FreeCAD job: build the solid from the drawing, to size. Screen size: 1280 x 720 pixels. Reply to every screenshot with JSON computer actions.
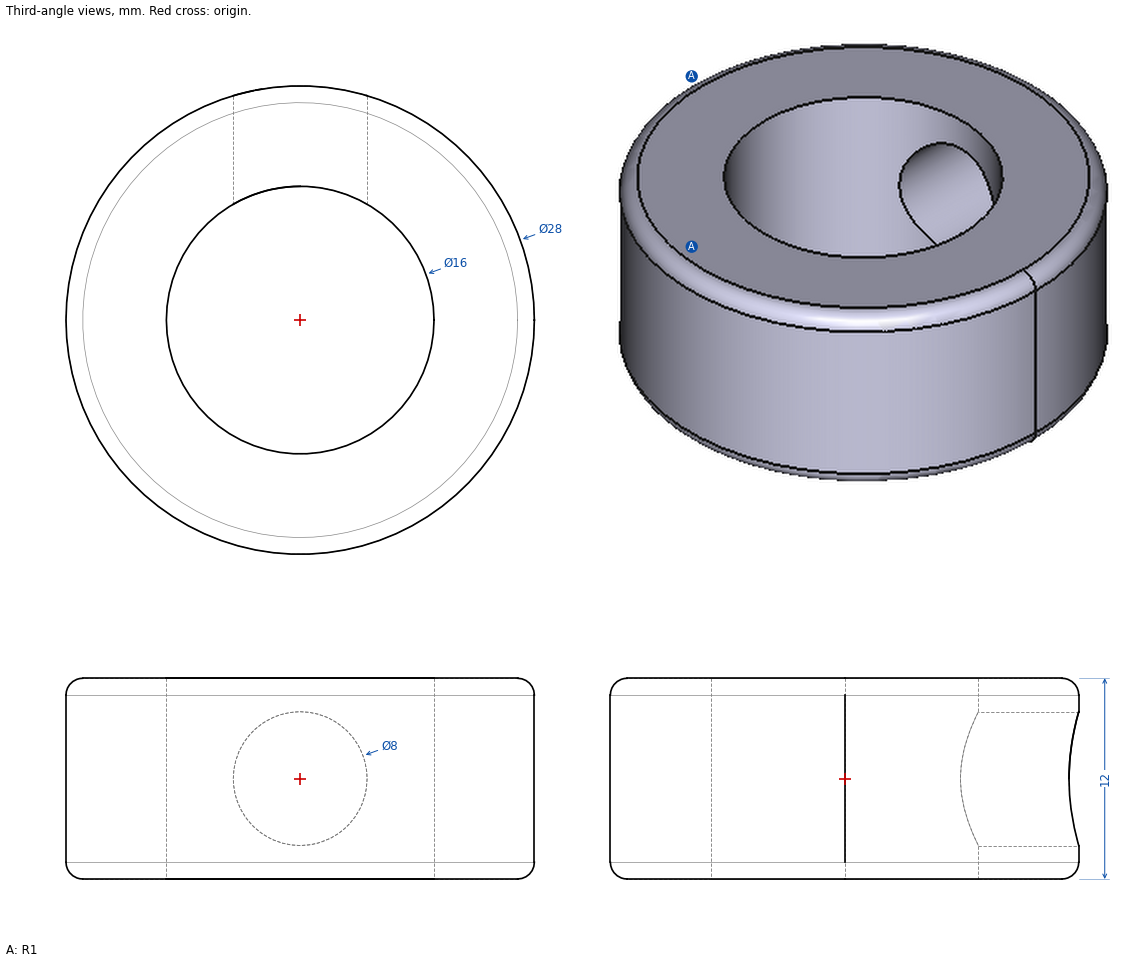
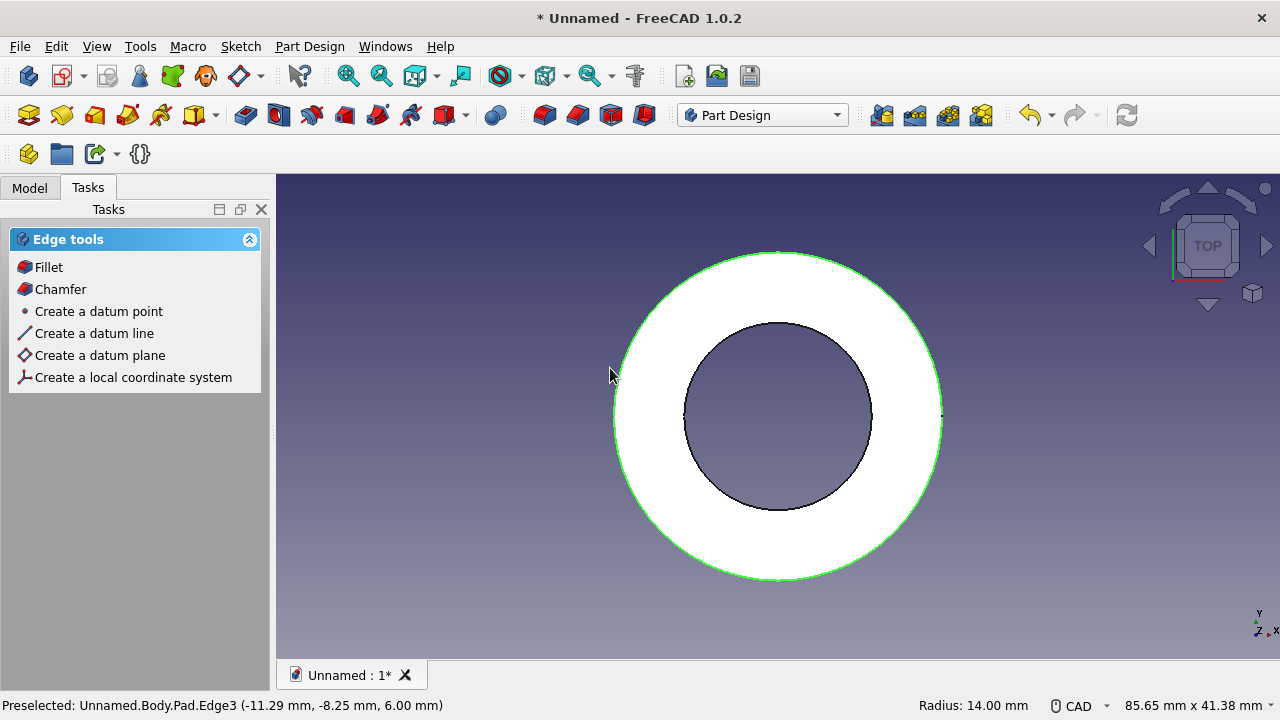
{"action": "key", "text": "1"}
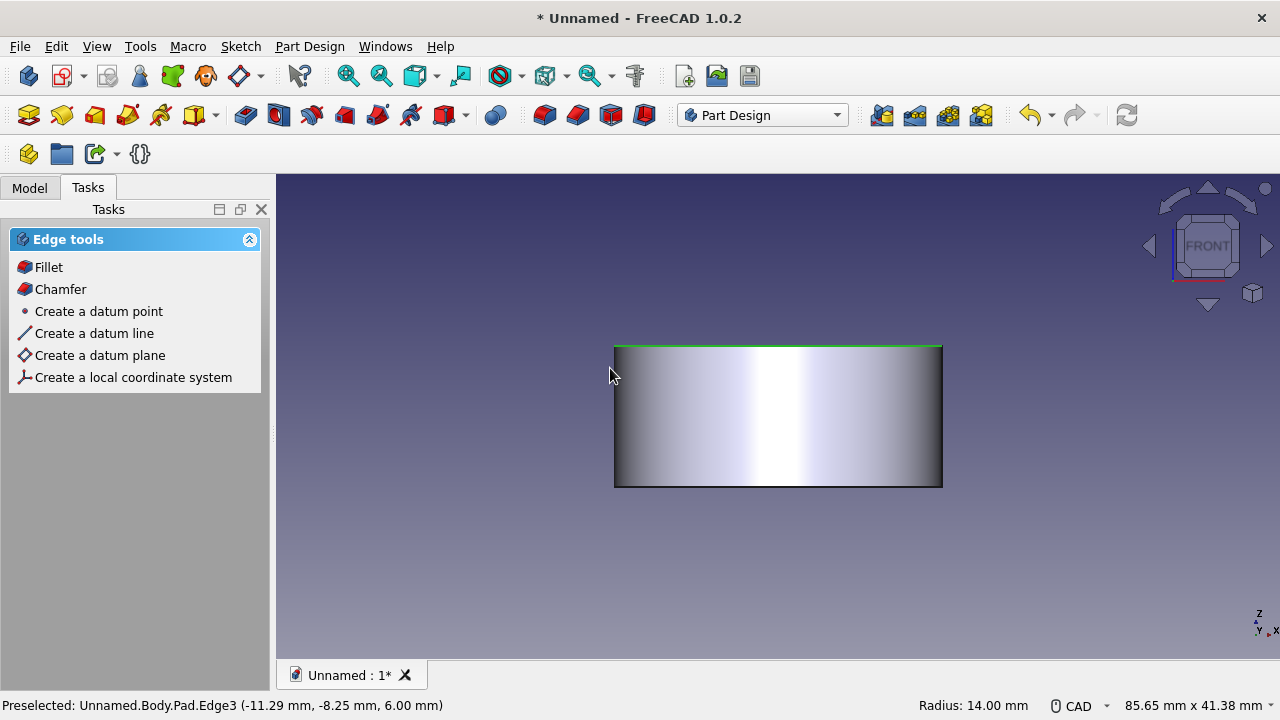
{"action": "key", "text": "v f"}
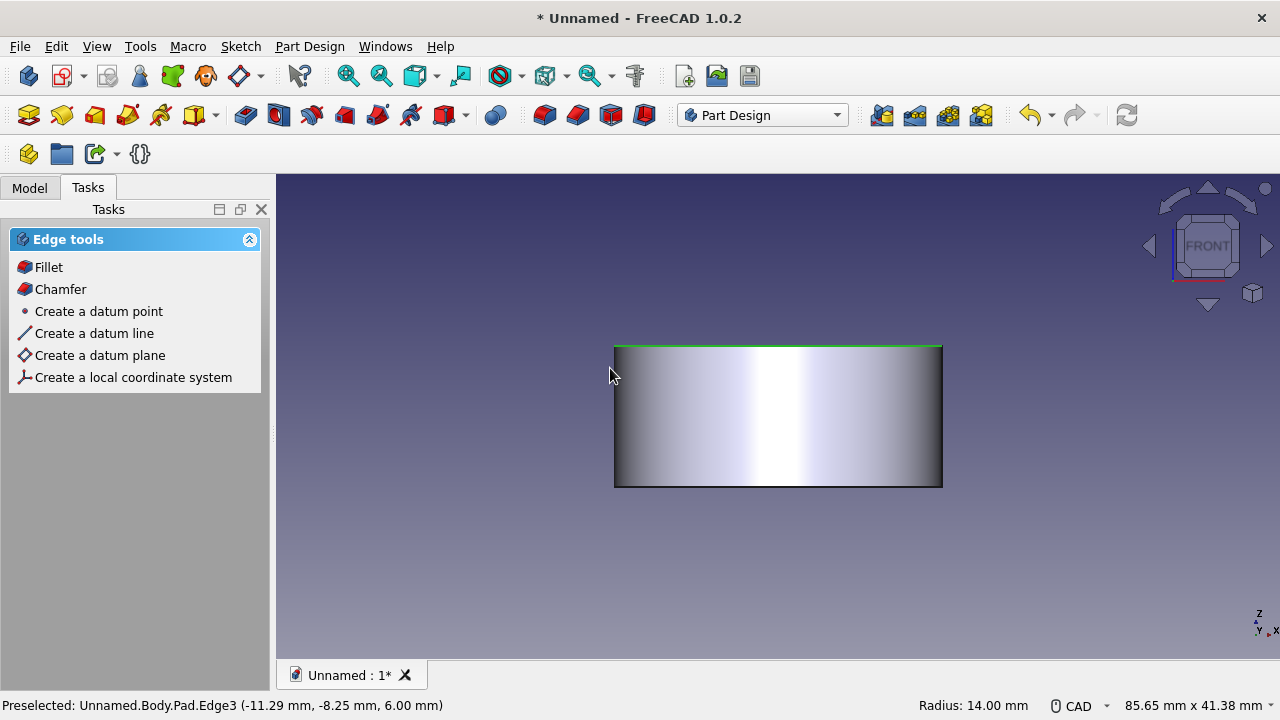
{"action": "left_click", "coordinate": [645, 486], "text": "ctrl"}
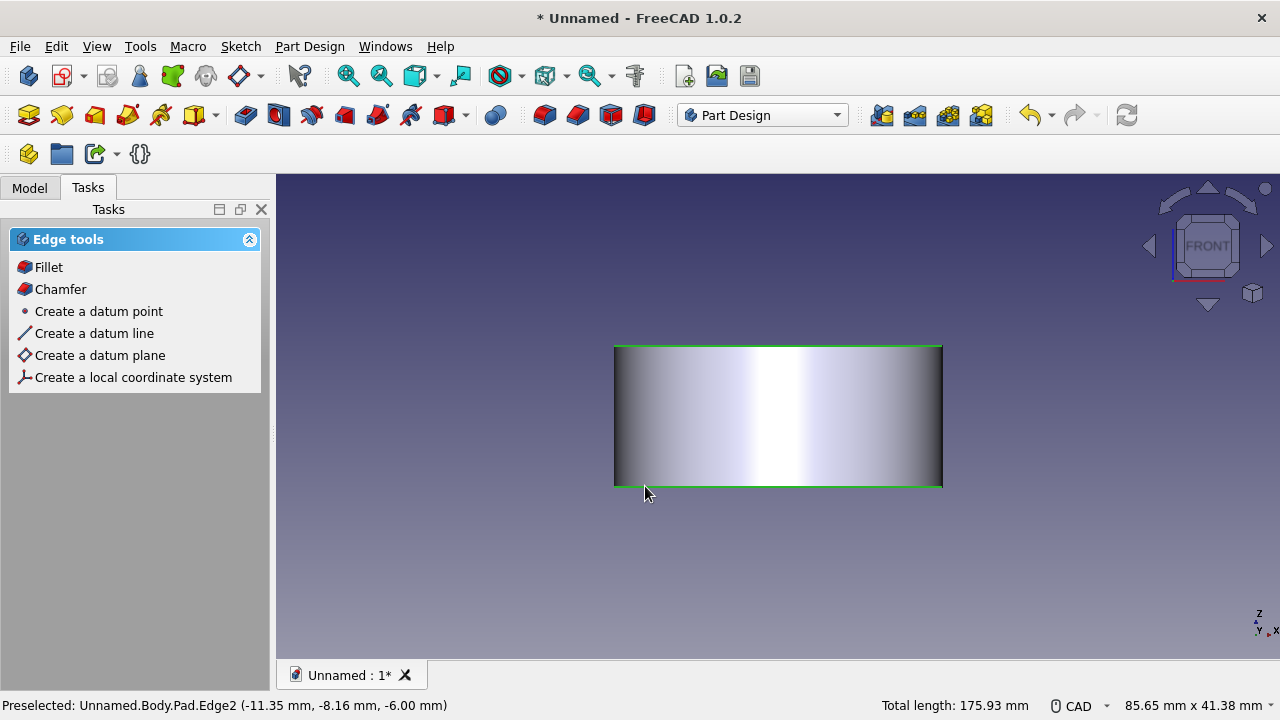
{"action": "left_click", "coordinate": [545, 116]}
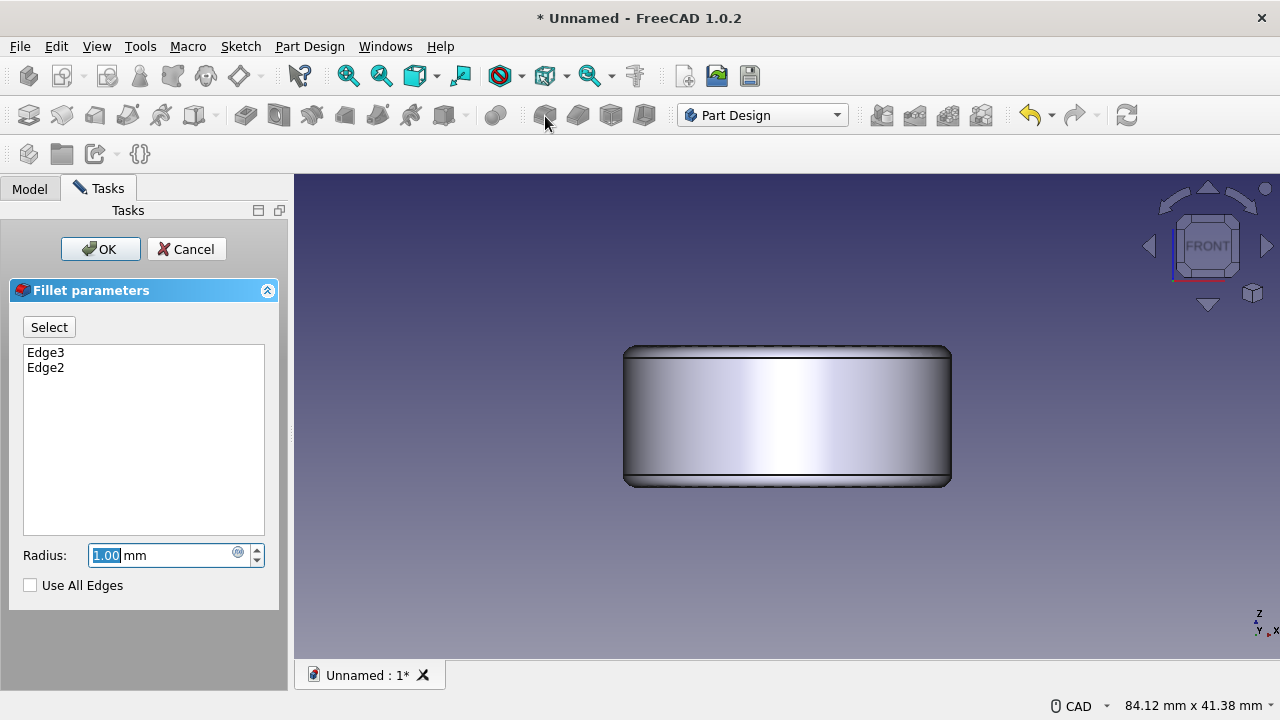
{"action": "type", "text": "1"}
{"action": "key", "text": "Tab"}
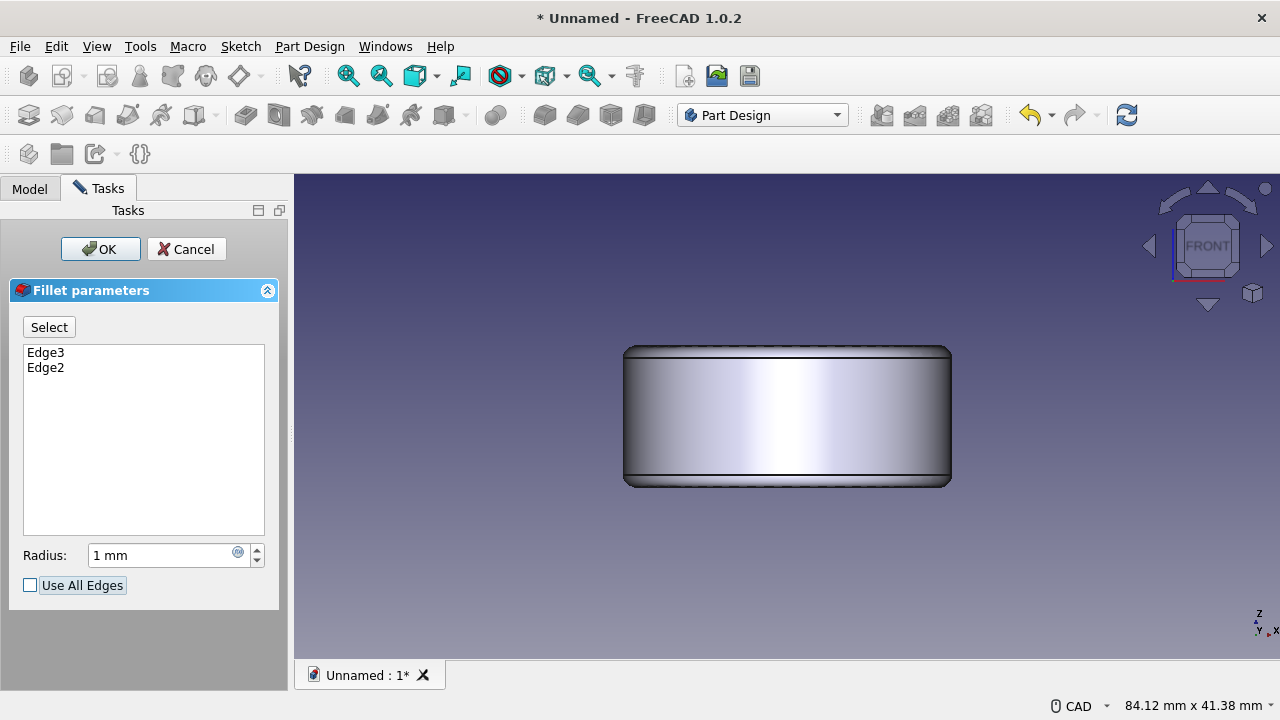
{"action": "left_click", "coordinate": [101, 249]}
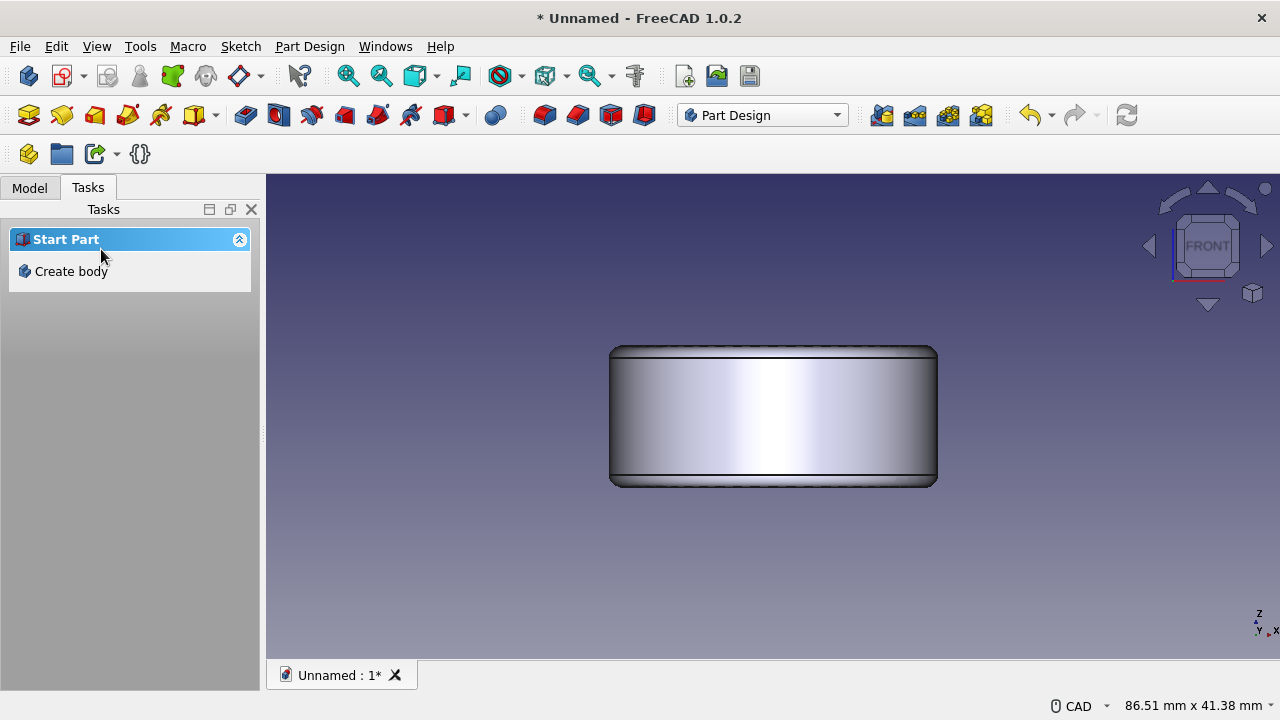
{"action": "key", "text": "v f"}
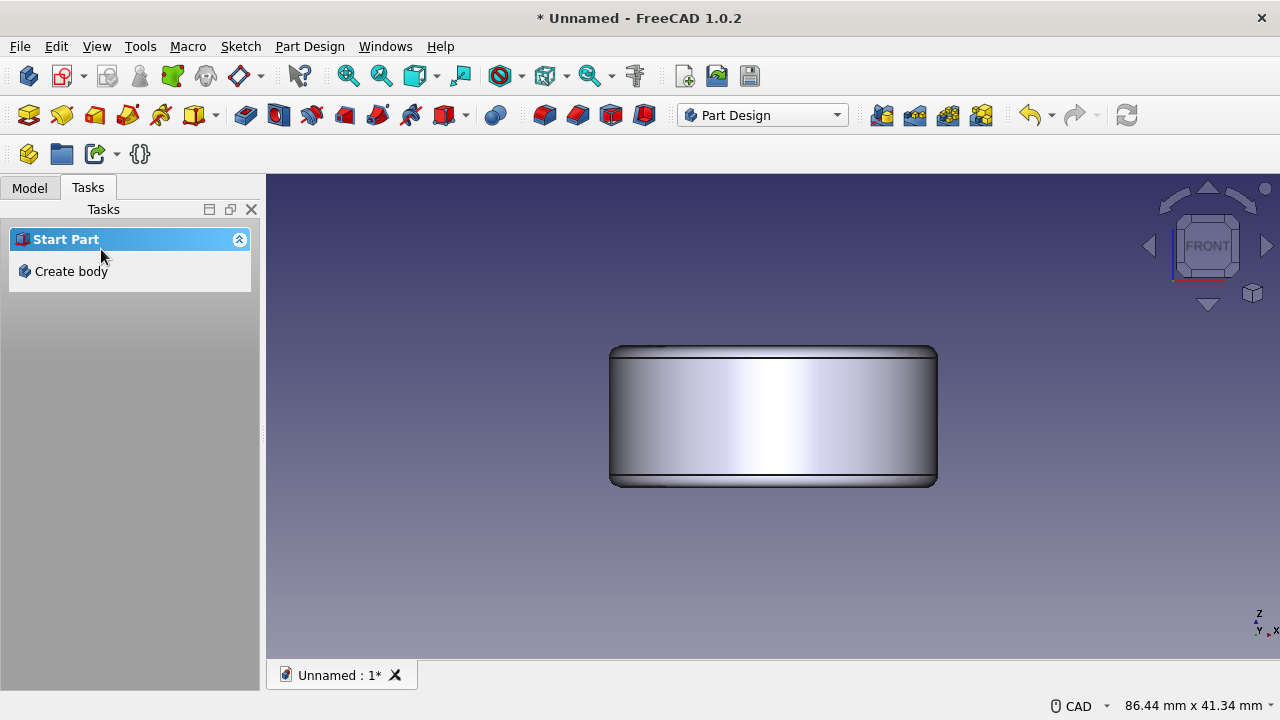
{"action": "left_click", "coordinate": [62, 76]}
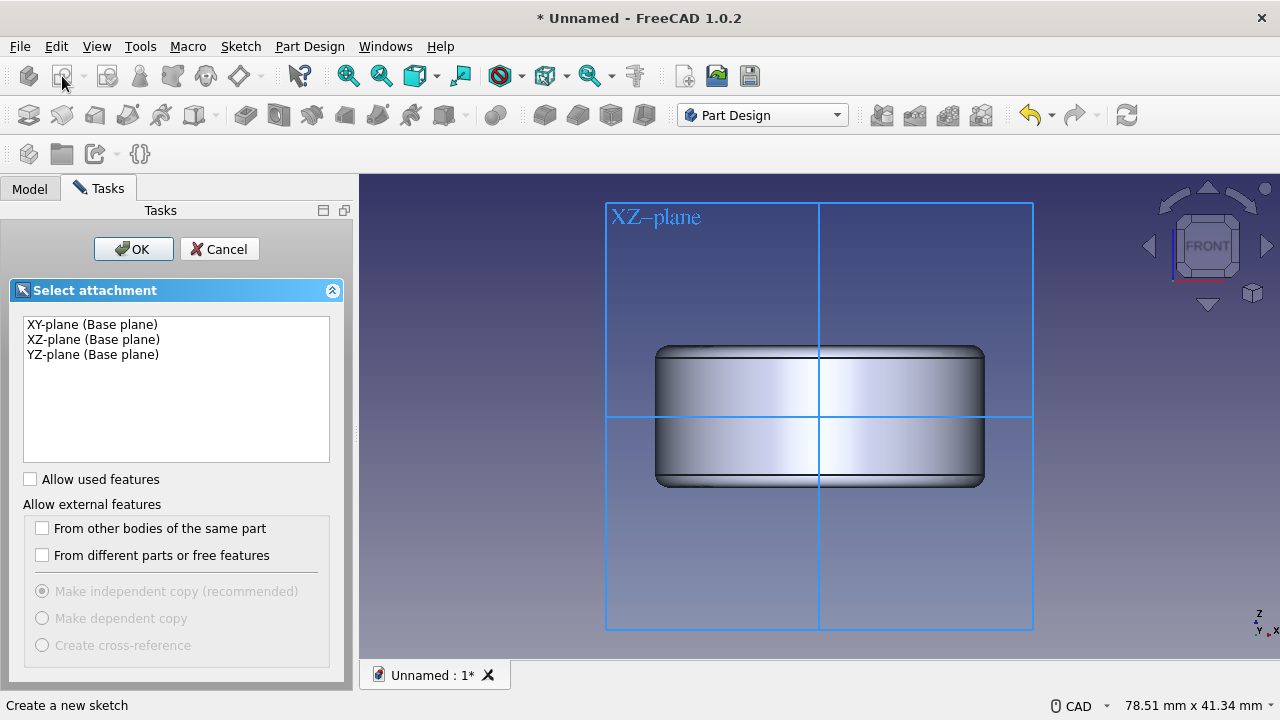
{"action": "left_click", "coordinate": [84, 340]}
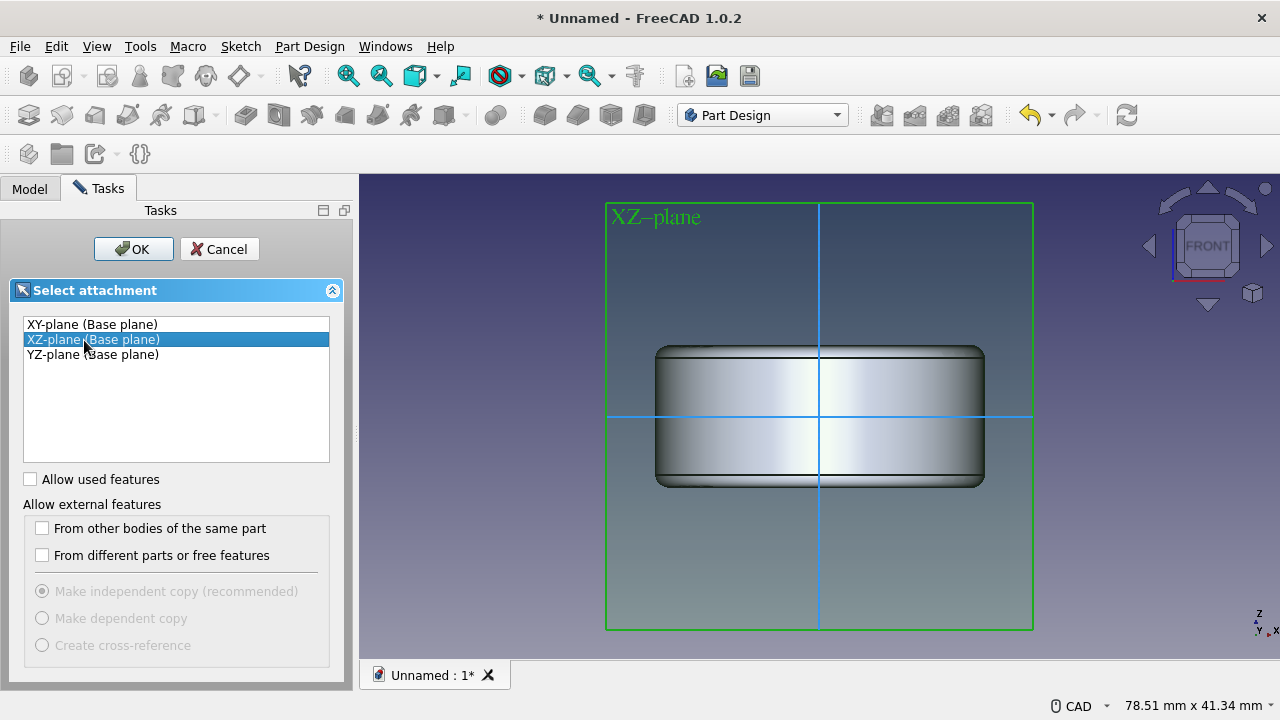
{"action": "left_click", "coordinate": [134, 249]}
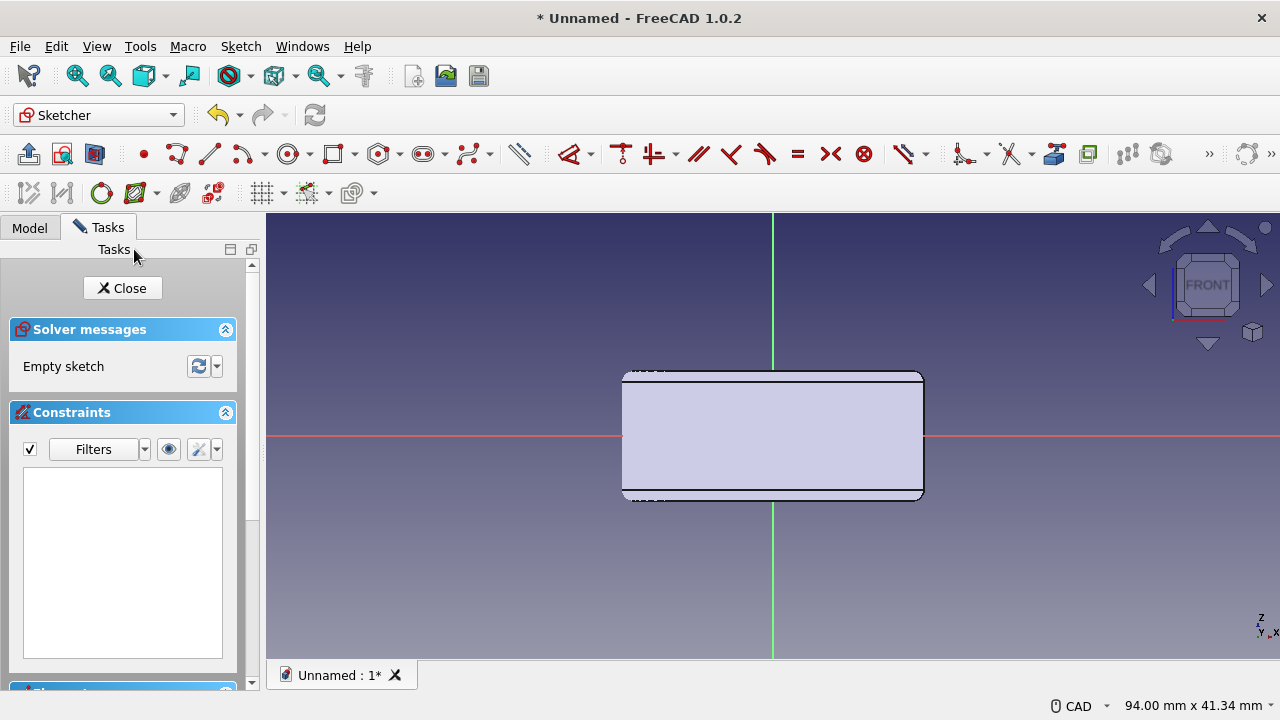
{"action": "key", "text": "q s"}